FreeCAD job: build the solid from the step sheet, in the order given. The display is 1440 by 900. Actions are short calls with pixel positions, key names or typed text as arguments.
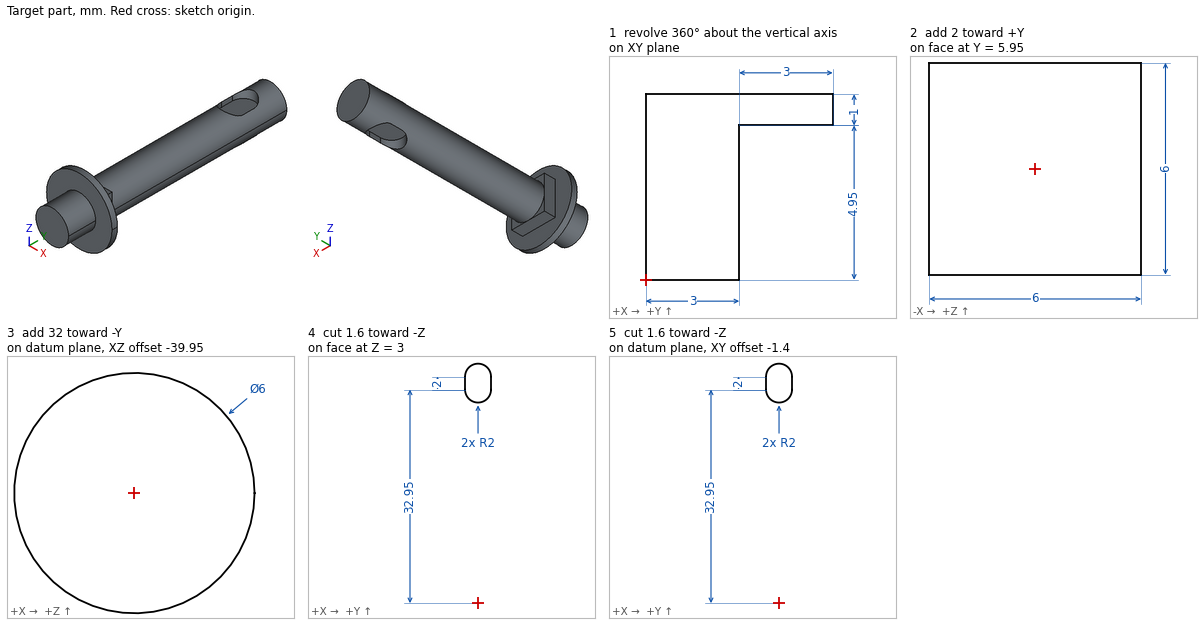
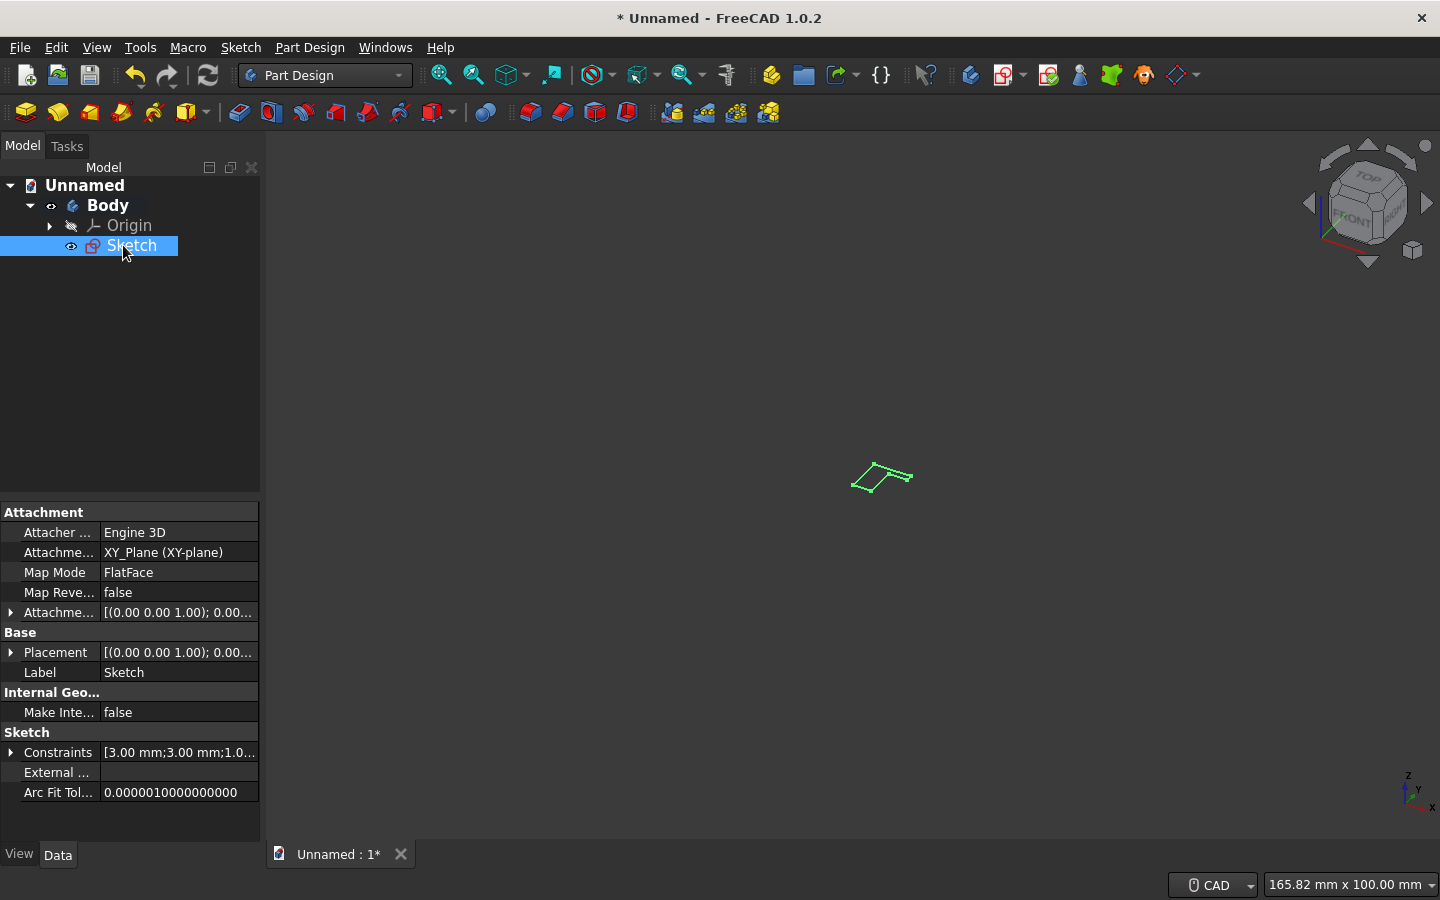
click(58, 112)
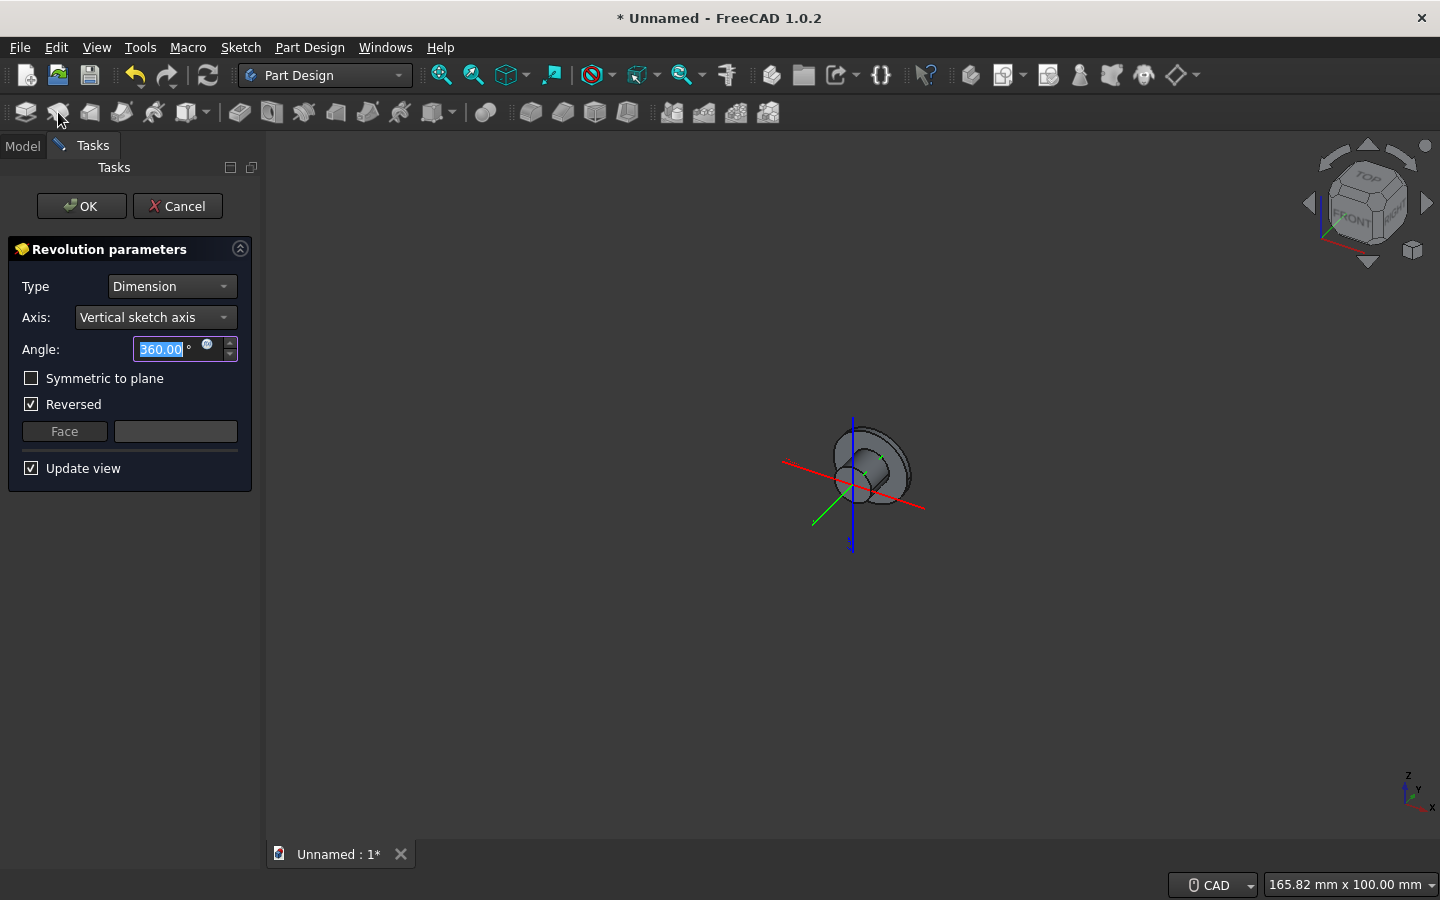
click(82, 206)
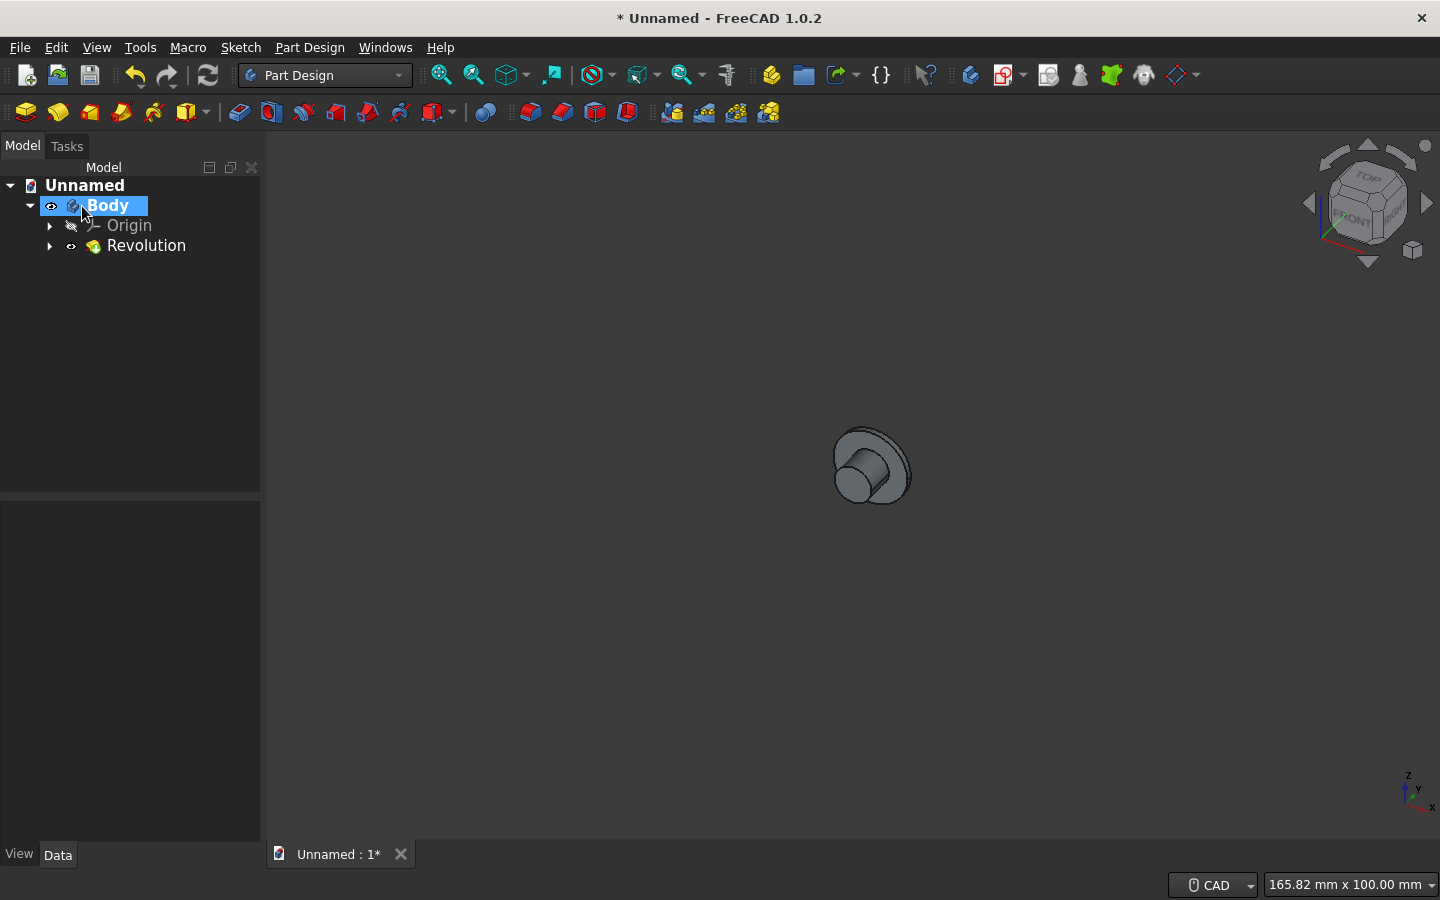
click(442, 76)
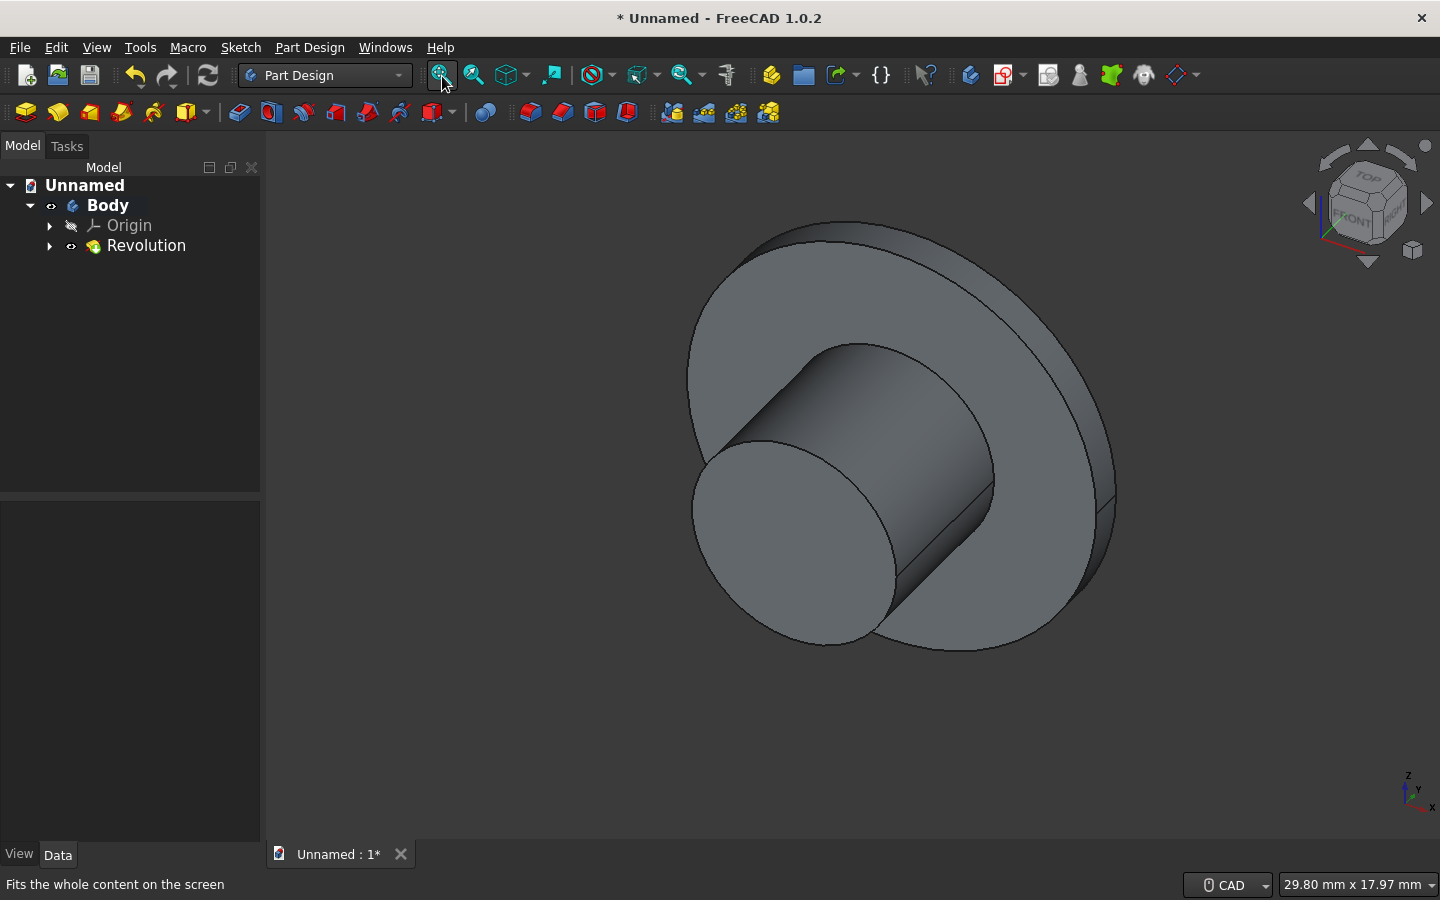
key(4)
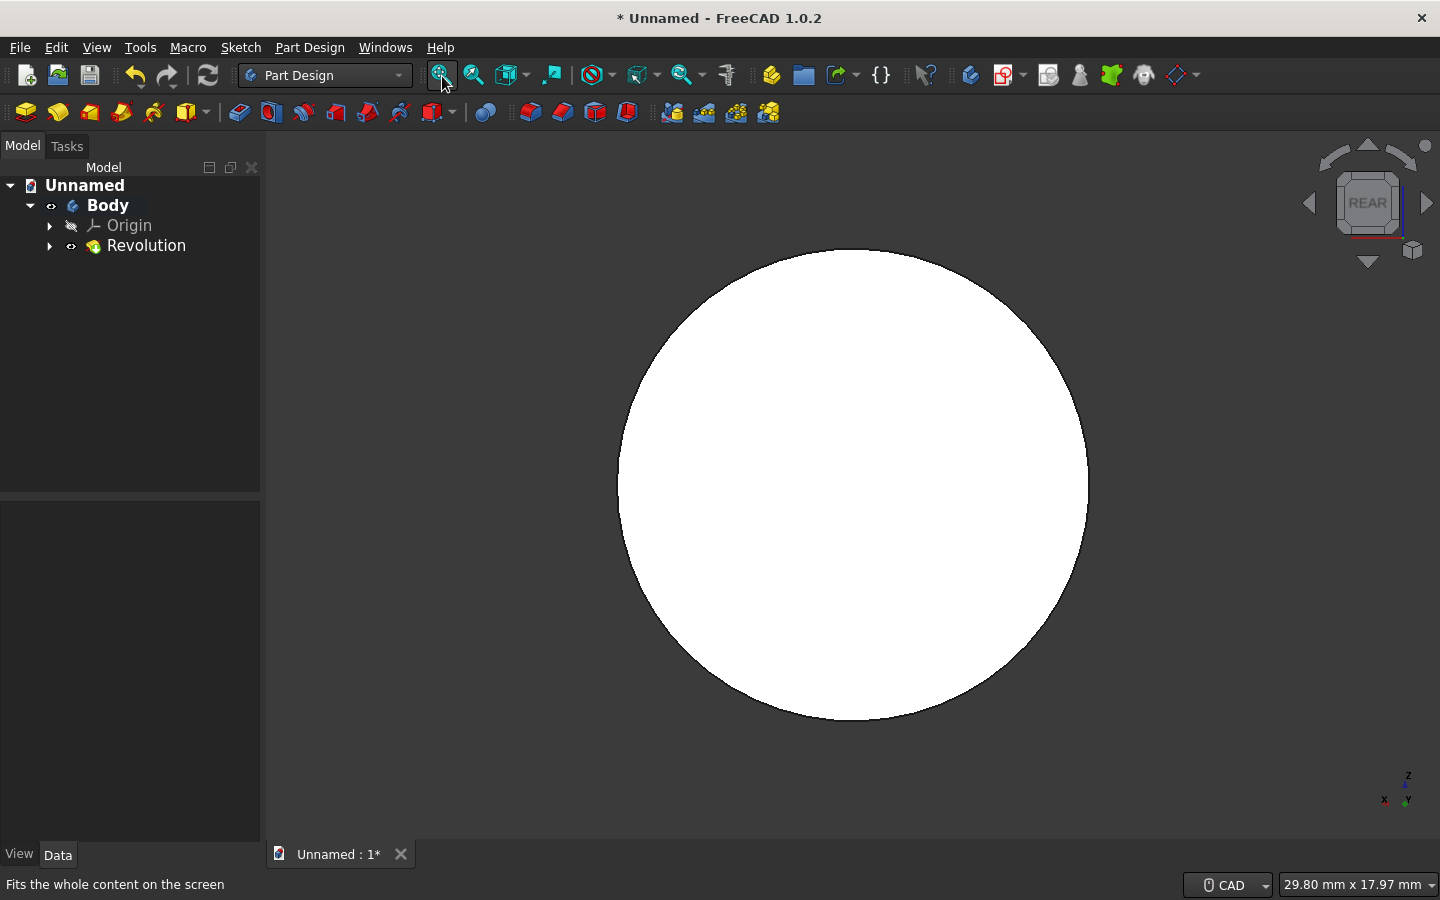
click(853, 484)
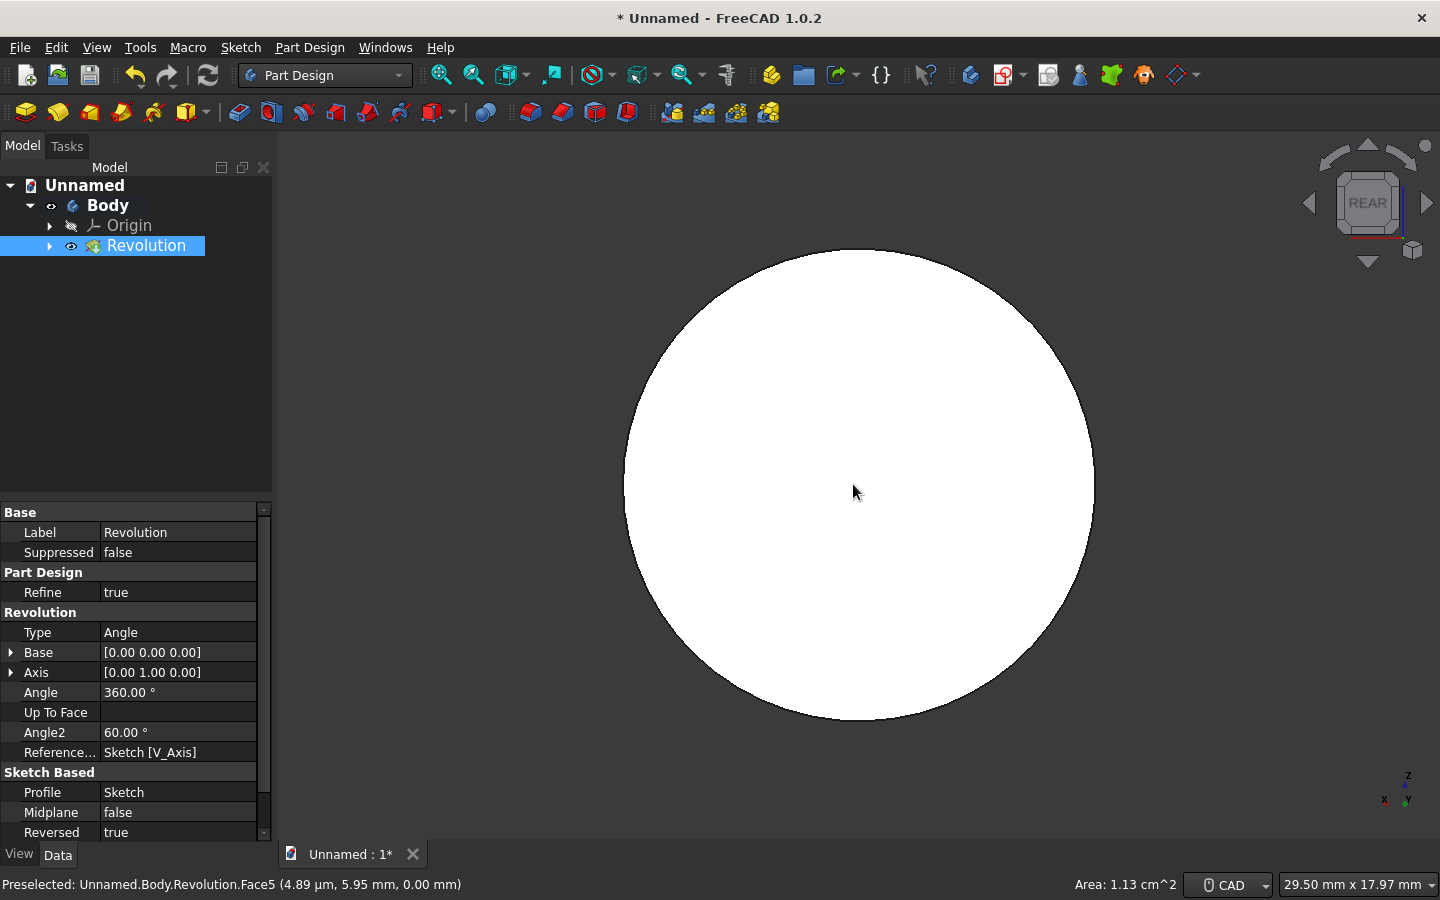
click(1004, 76)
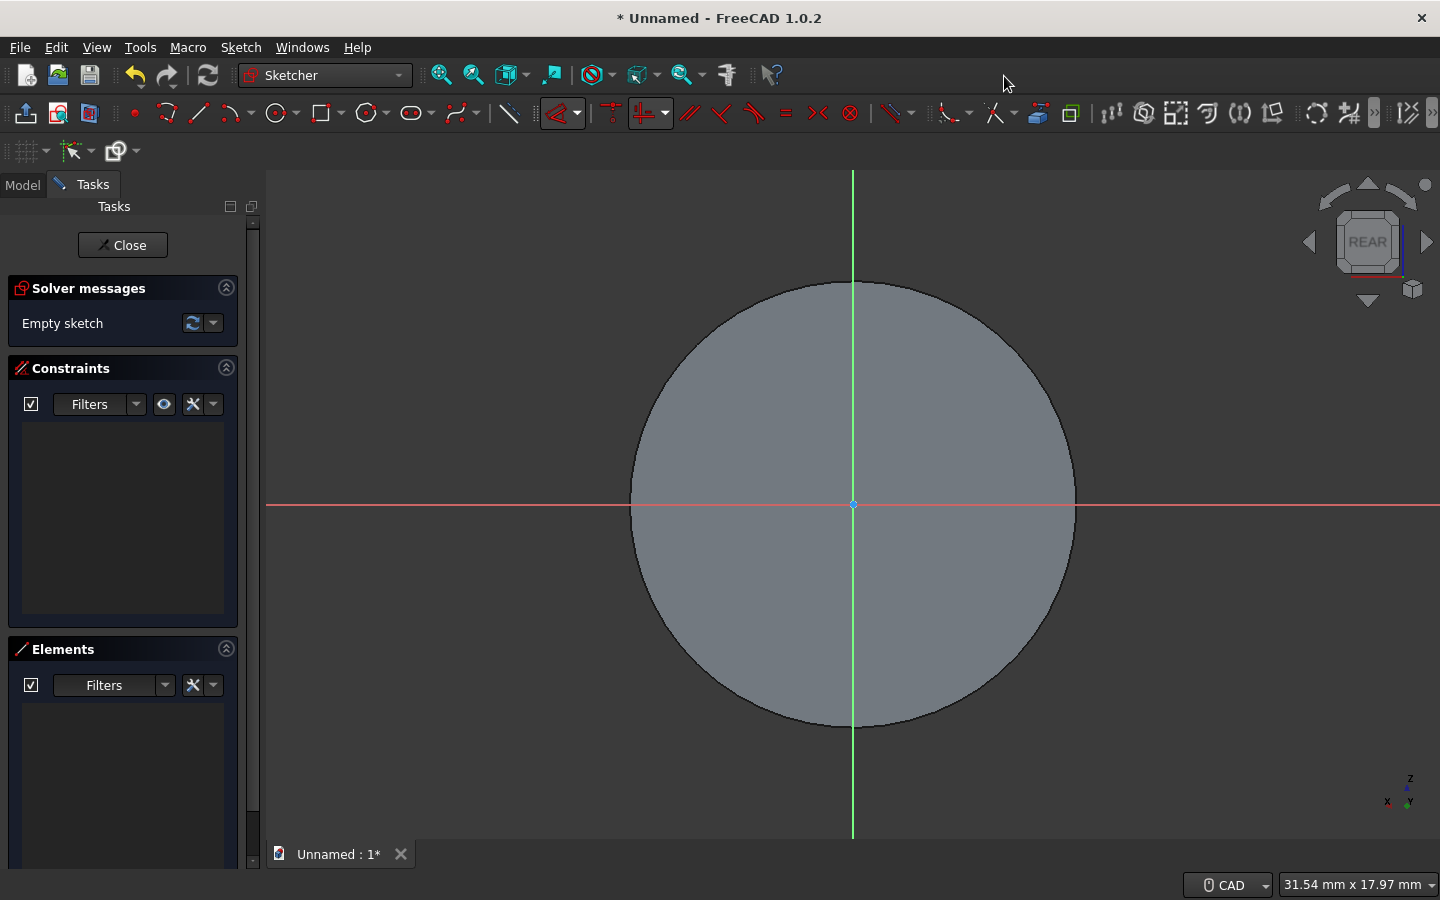
scroll(937, 504, up, 3)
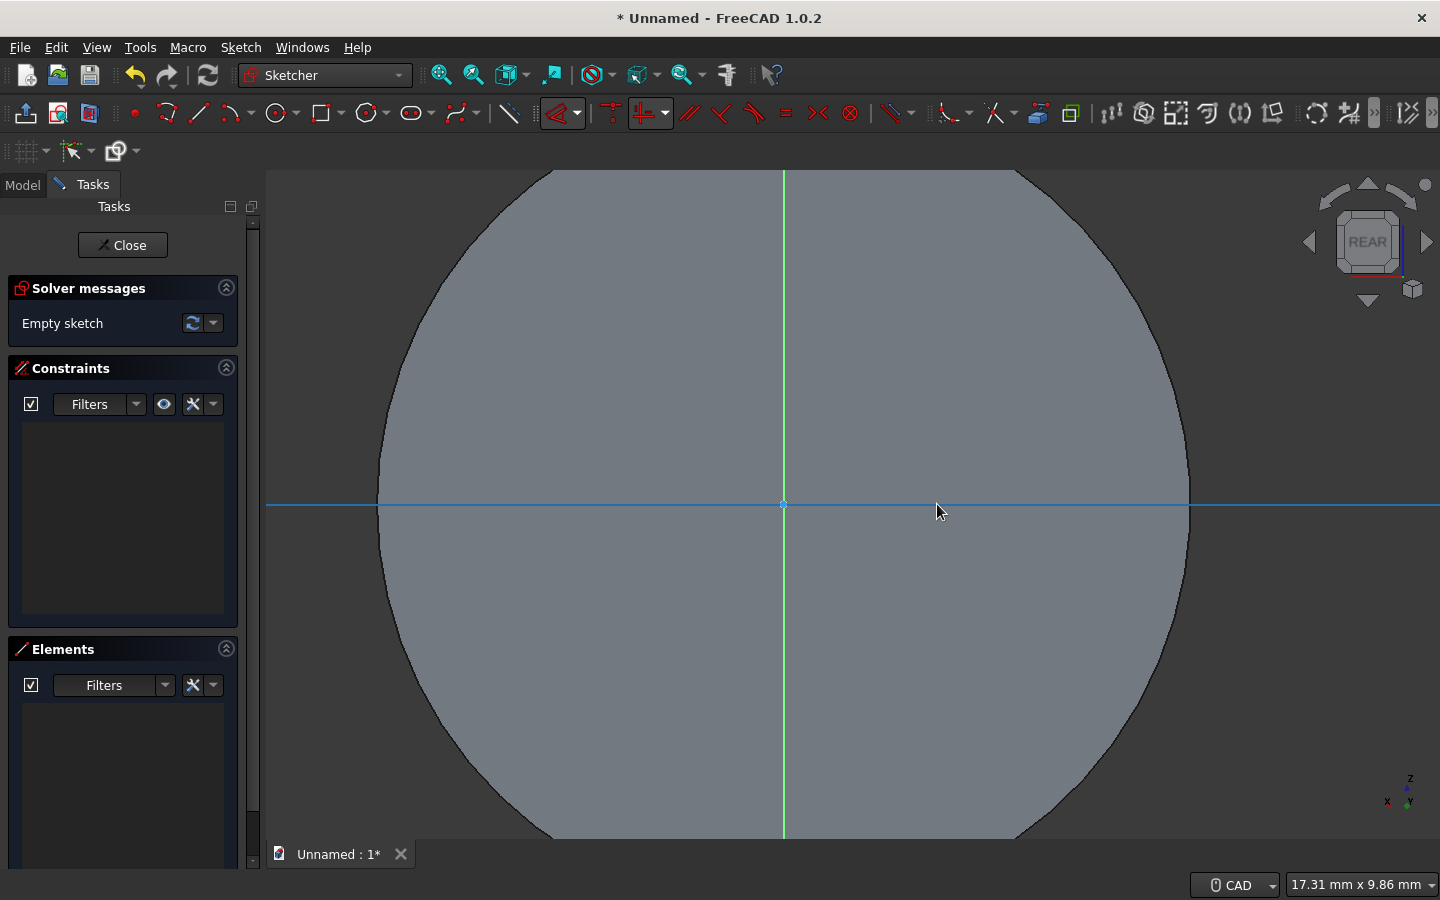
key(g)
key(v)